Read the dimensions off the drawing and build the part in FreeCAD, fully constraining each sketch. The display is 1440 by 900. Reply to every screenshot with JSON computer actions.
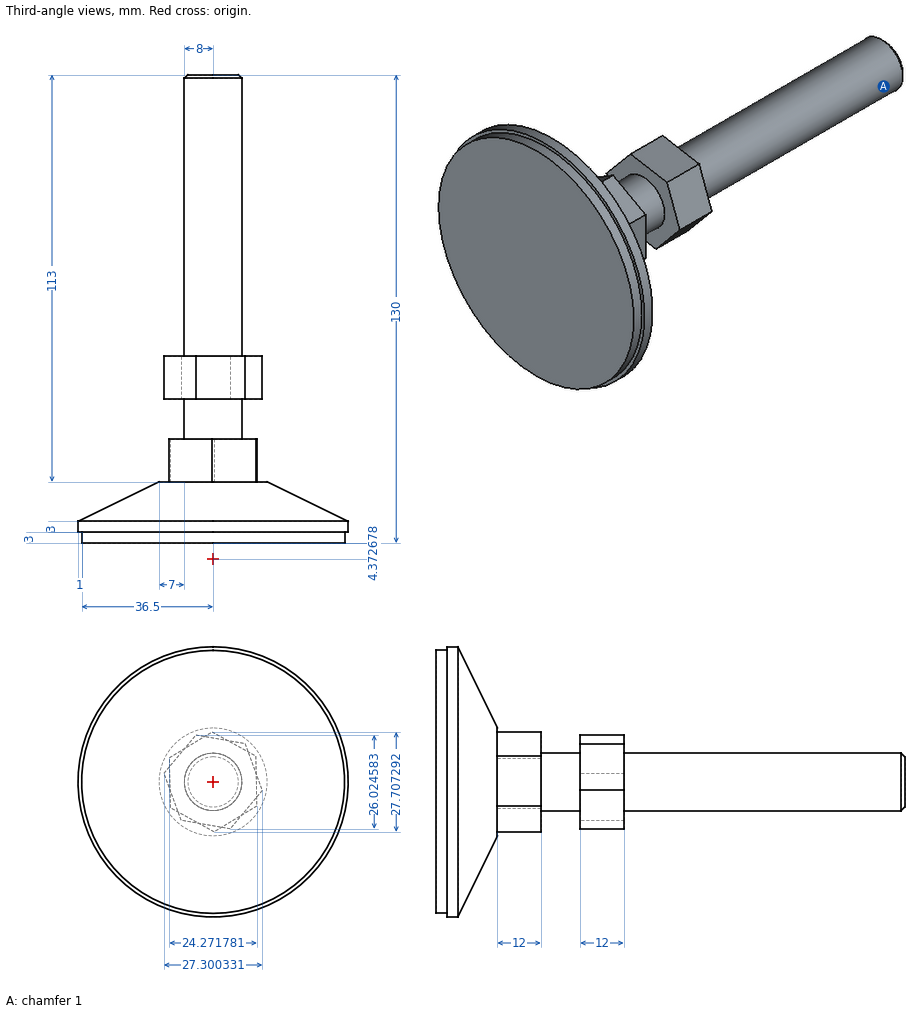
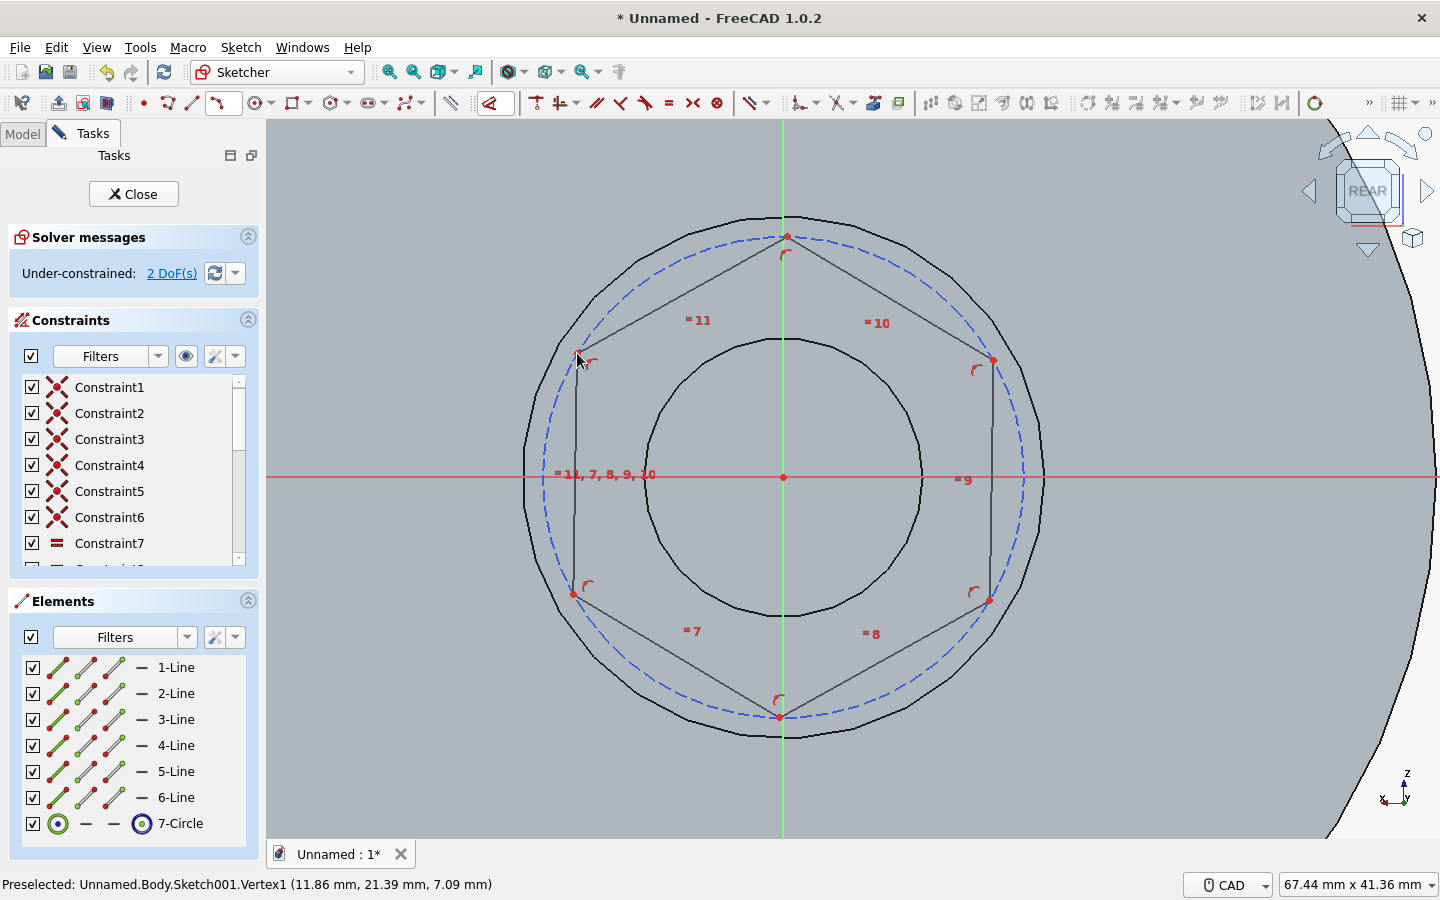
{"action": "left_click", "coordinate": [573, 594]}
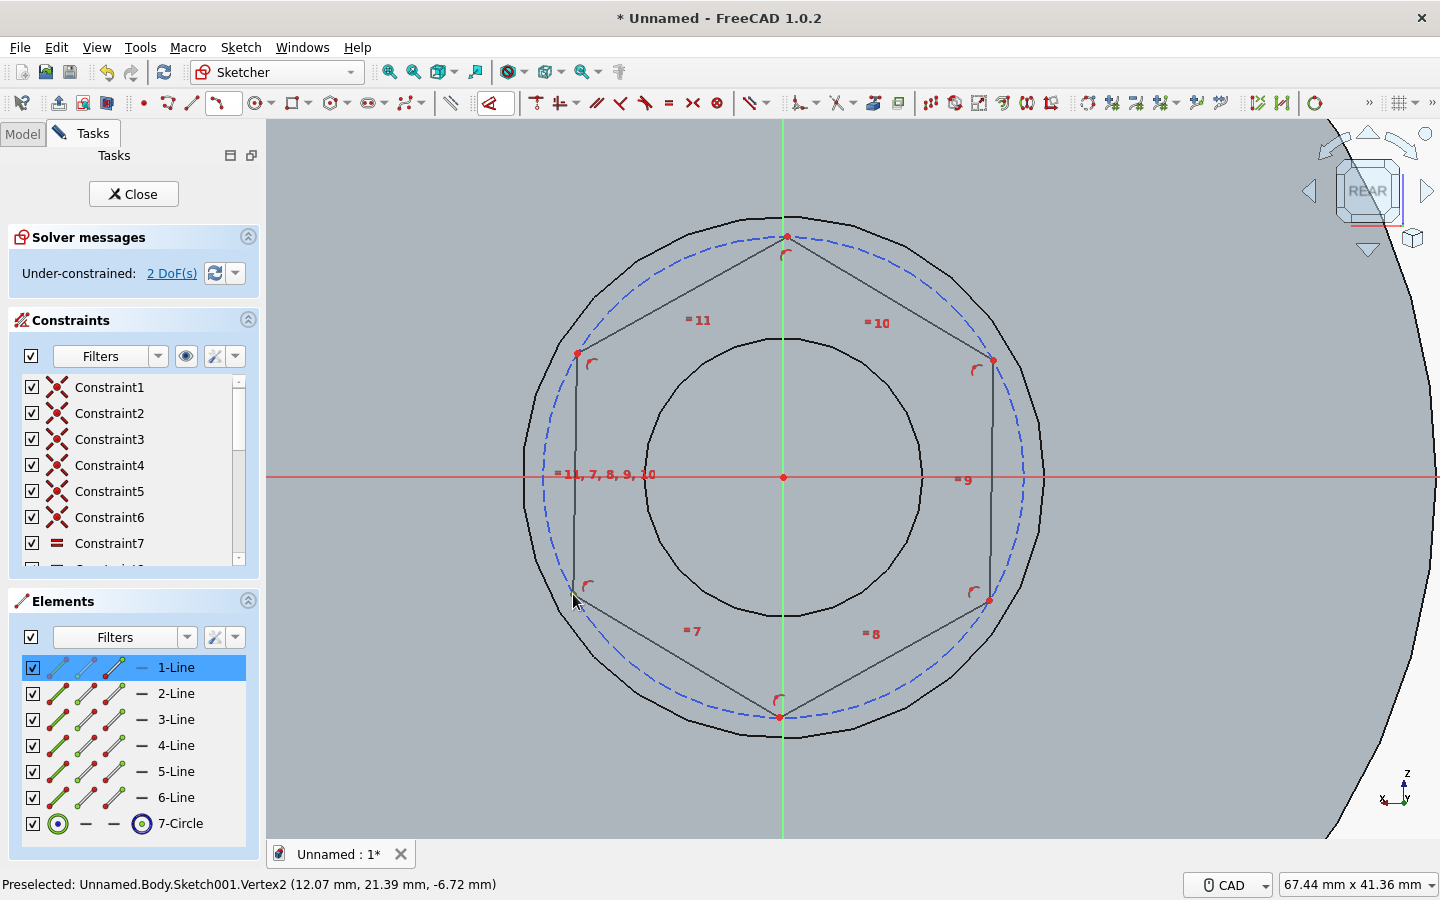
{"action": "left_click", "coordinate": [994, 360]}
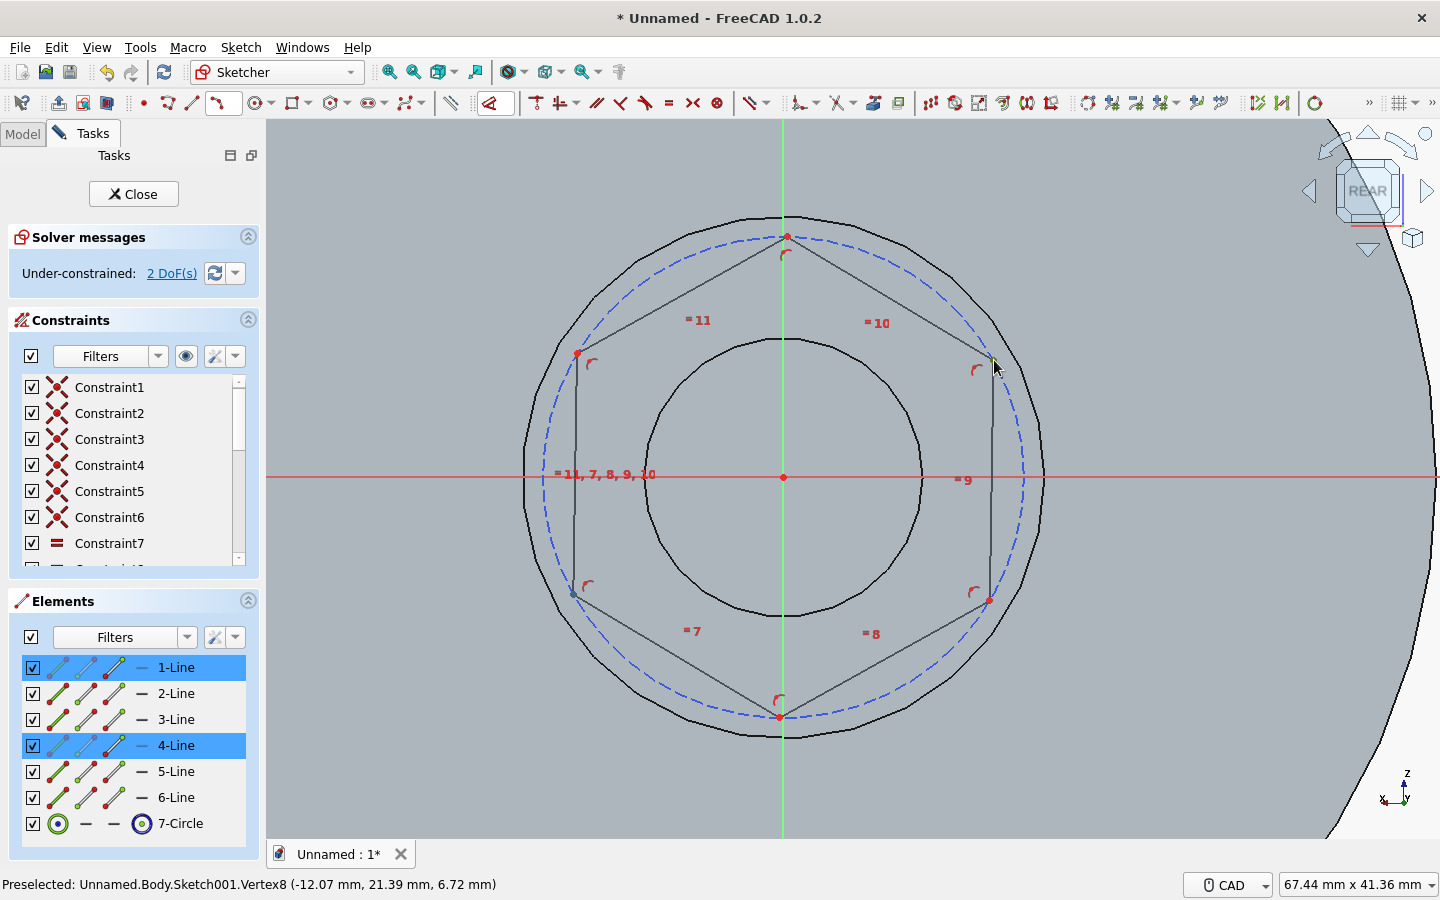
{"action": "left_click", "coordinate": [508, 104]}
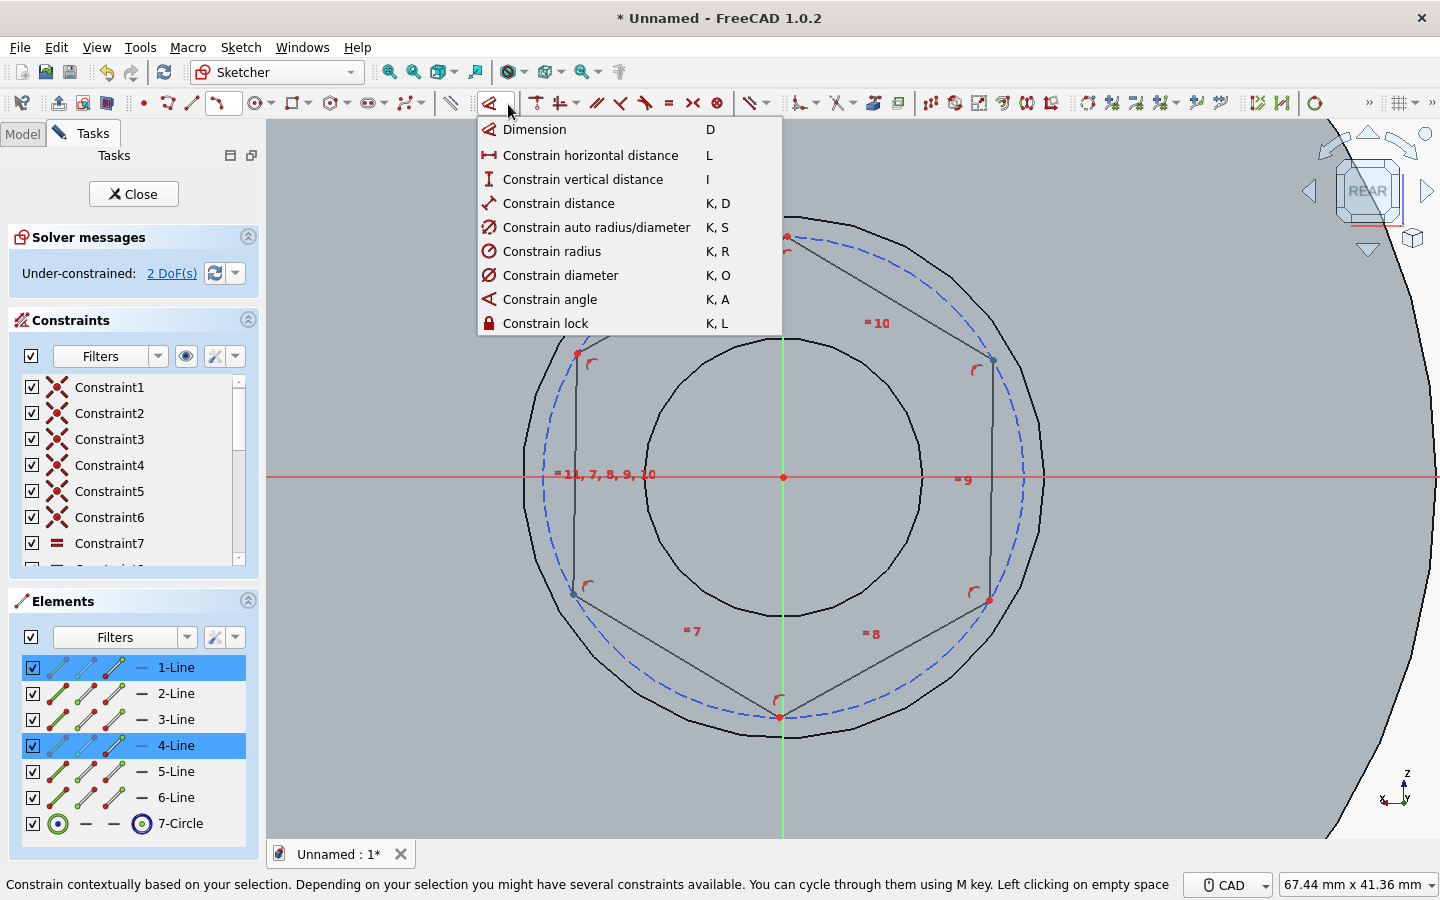
{"action": "left_click", "coordinate": [630, 155]}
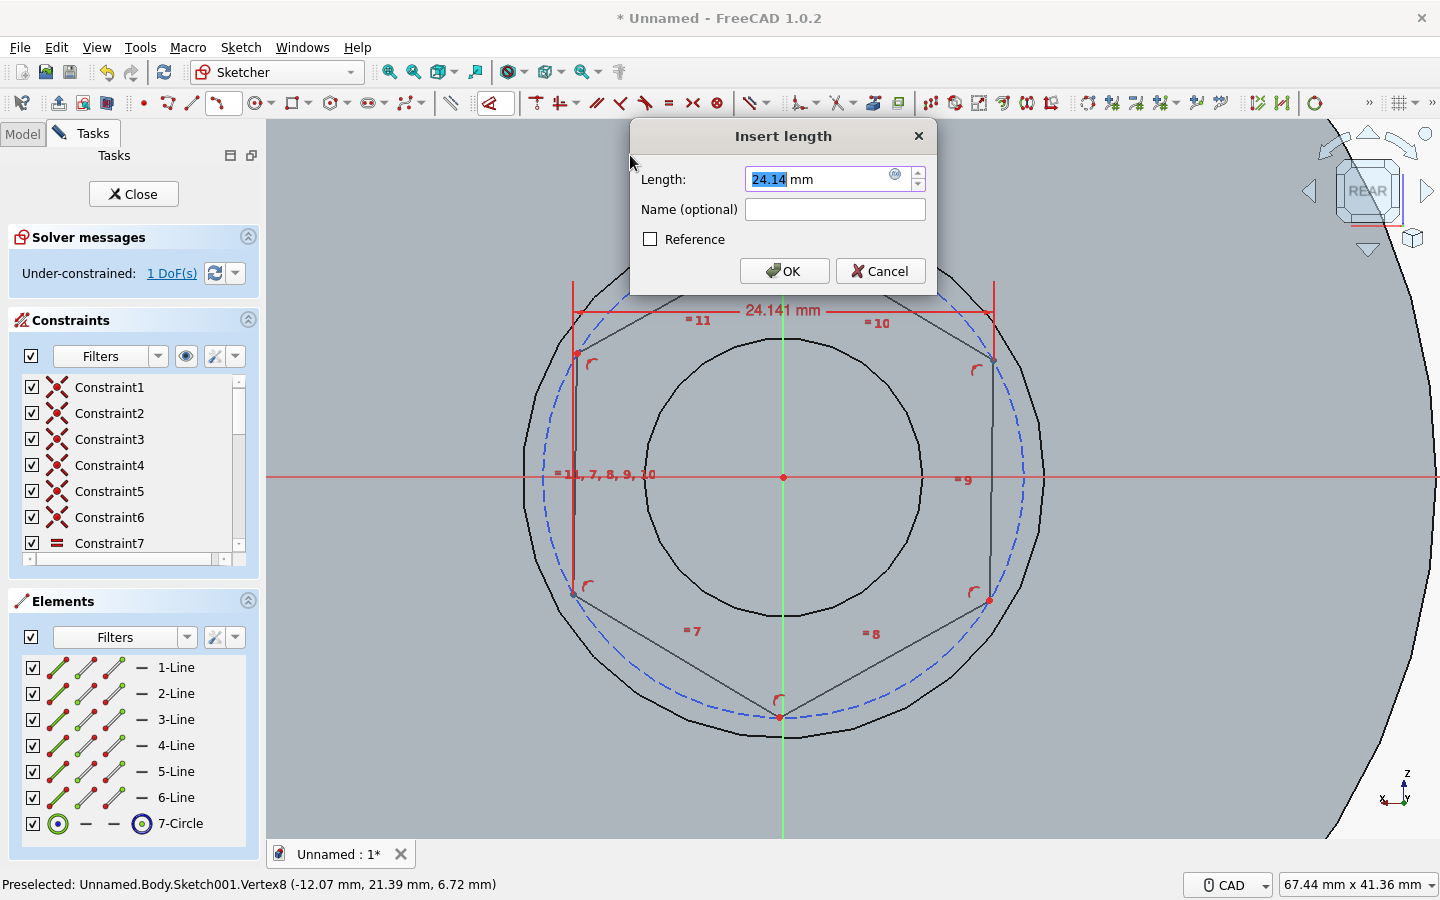
{"action": "type", "text": "24.271781"}
{"action": "key", "text": "Return"}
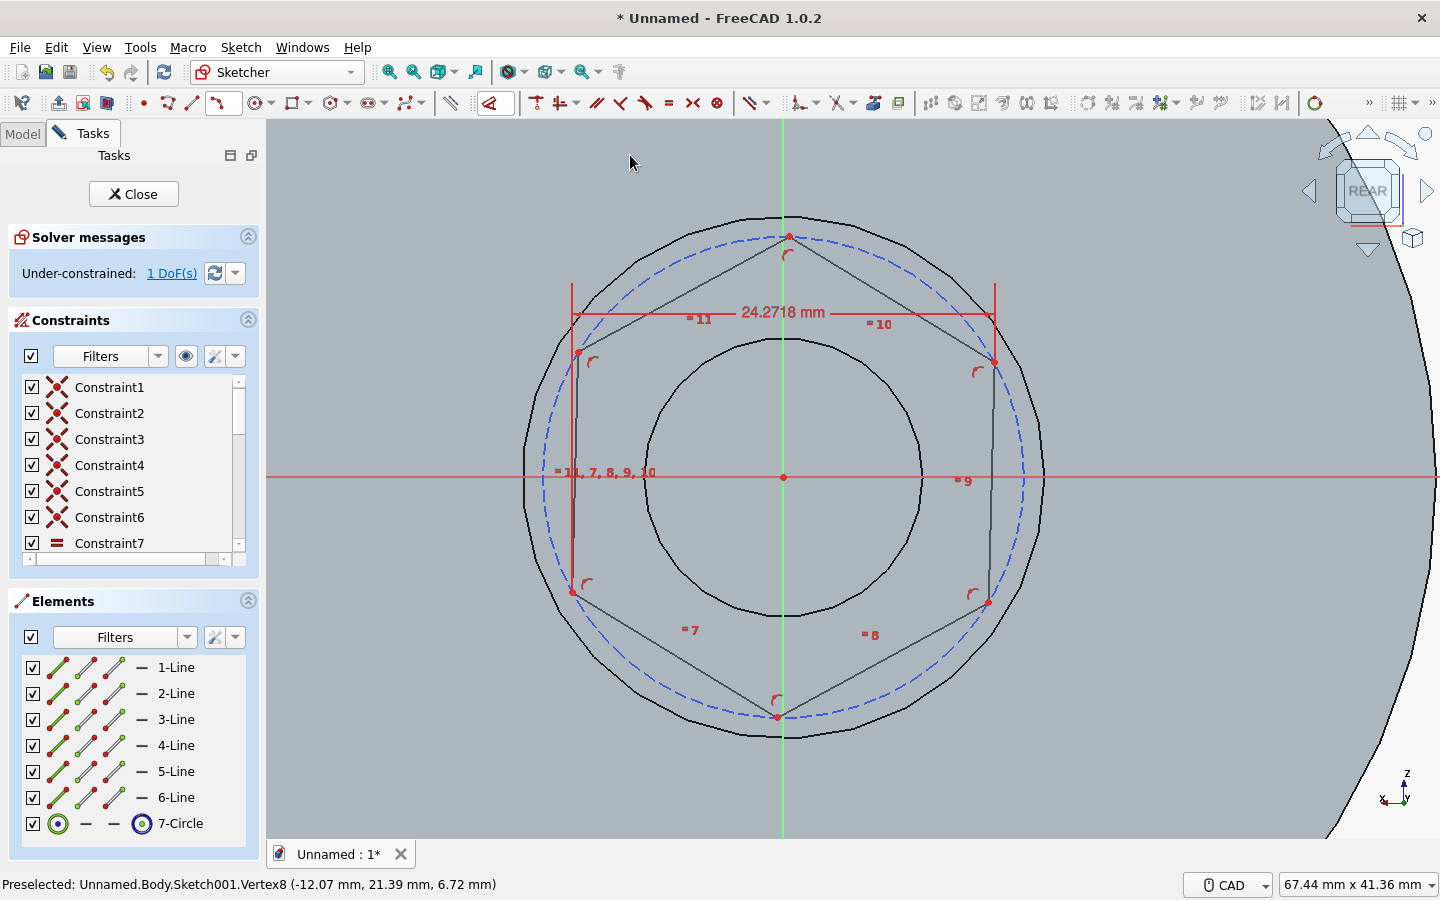
{"action": "left_click", "coordinate": [777, 718]}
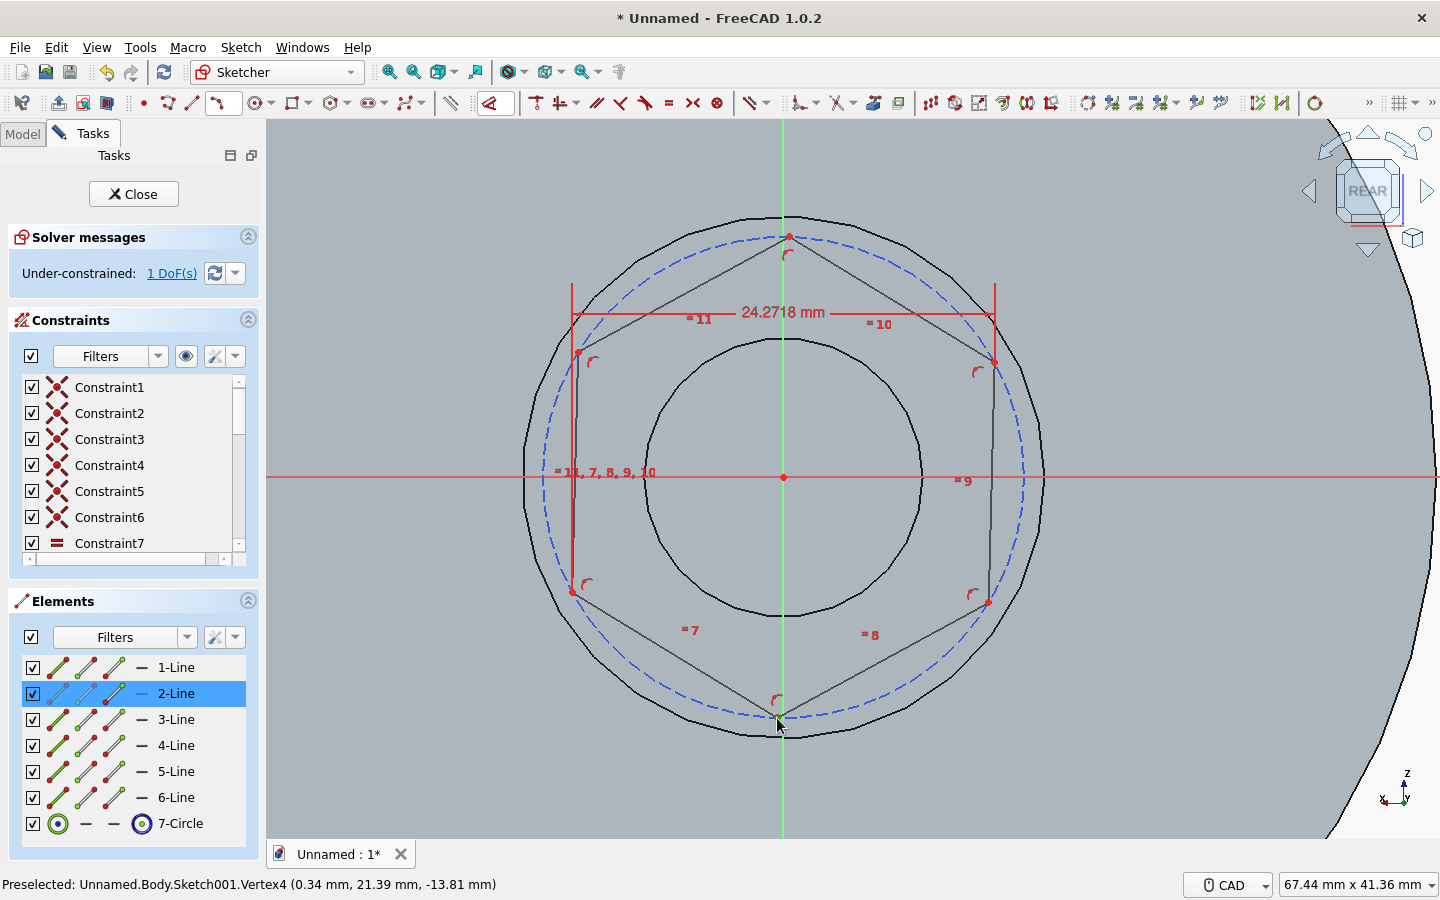
{"action": "left_click", "coordinate": [789, 237]}